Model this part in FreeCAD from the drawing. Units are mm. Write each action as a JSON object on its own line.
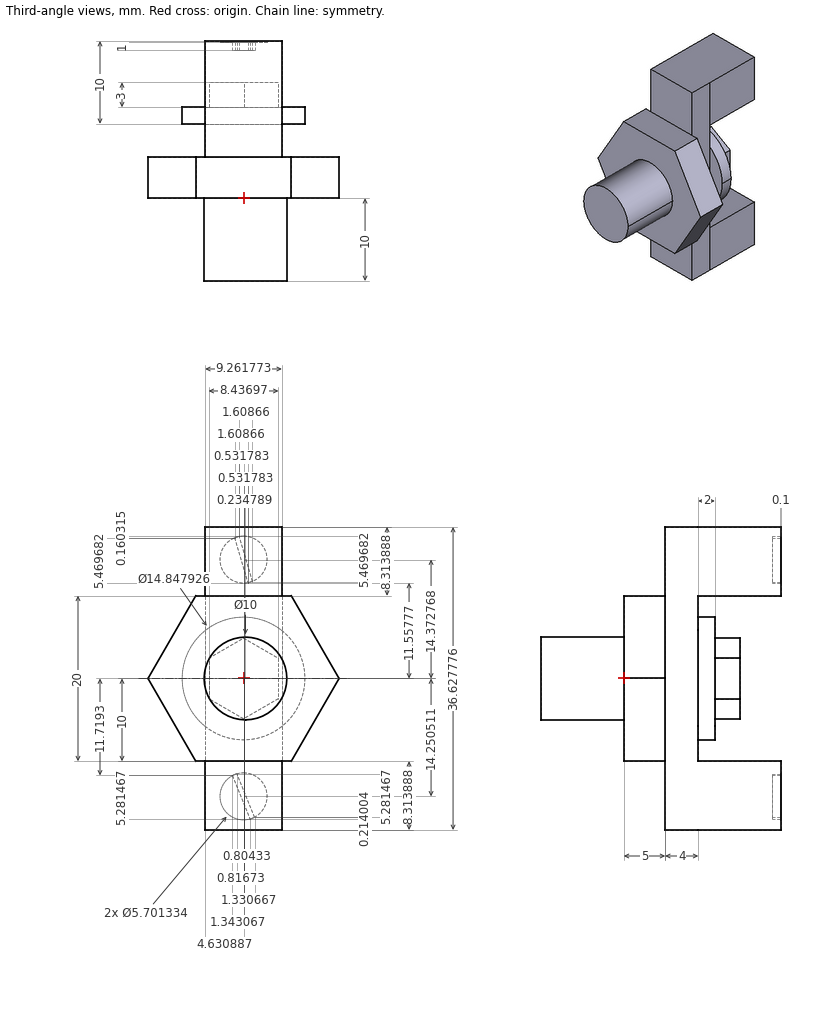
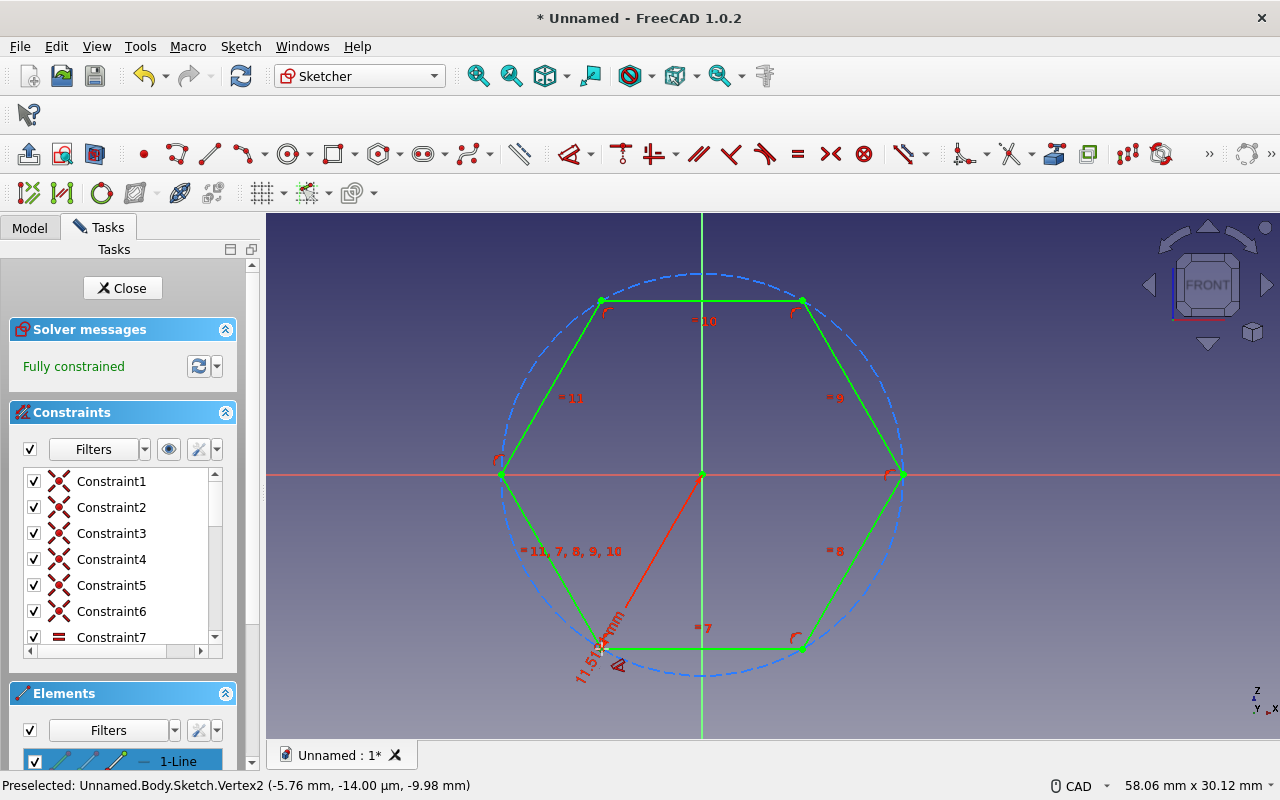
{"action": "left_click", "coordinate": [803, 301]}
{"action": "left_click", "coordinate": [837, 395]}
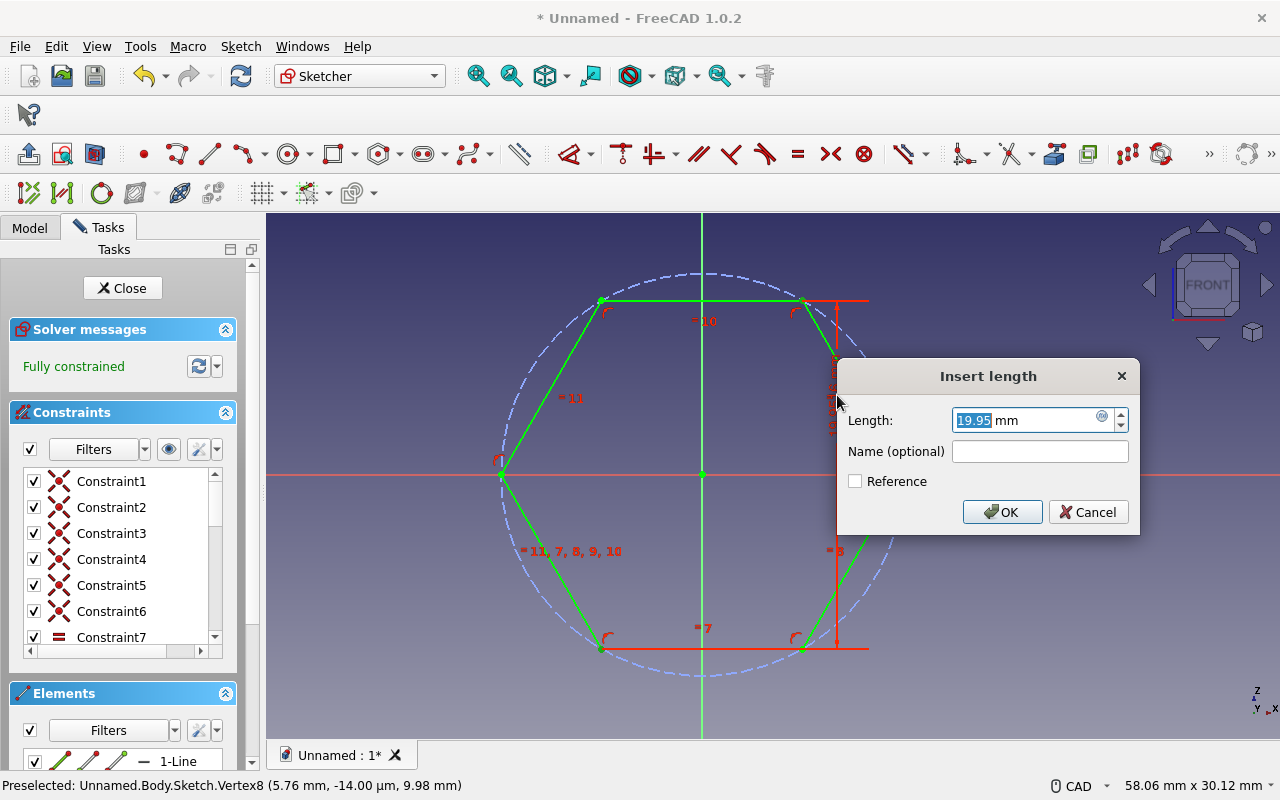
{"action": "type", "text": "20"}
{"action": "key", "text": "Return"}
{"action": "key", "text": "Escape"}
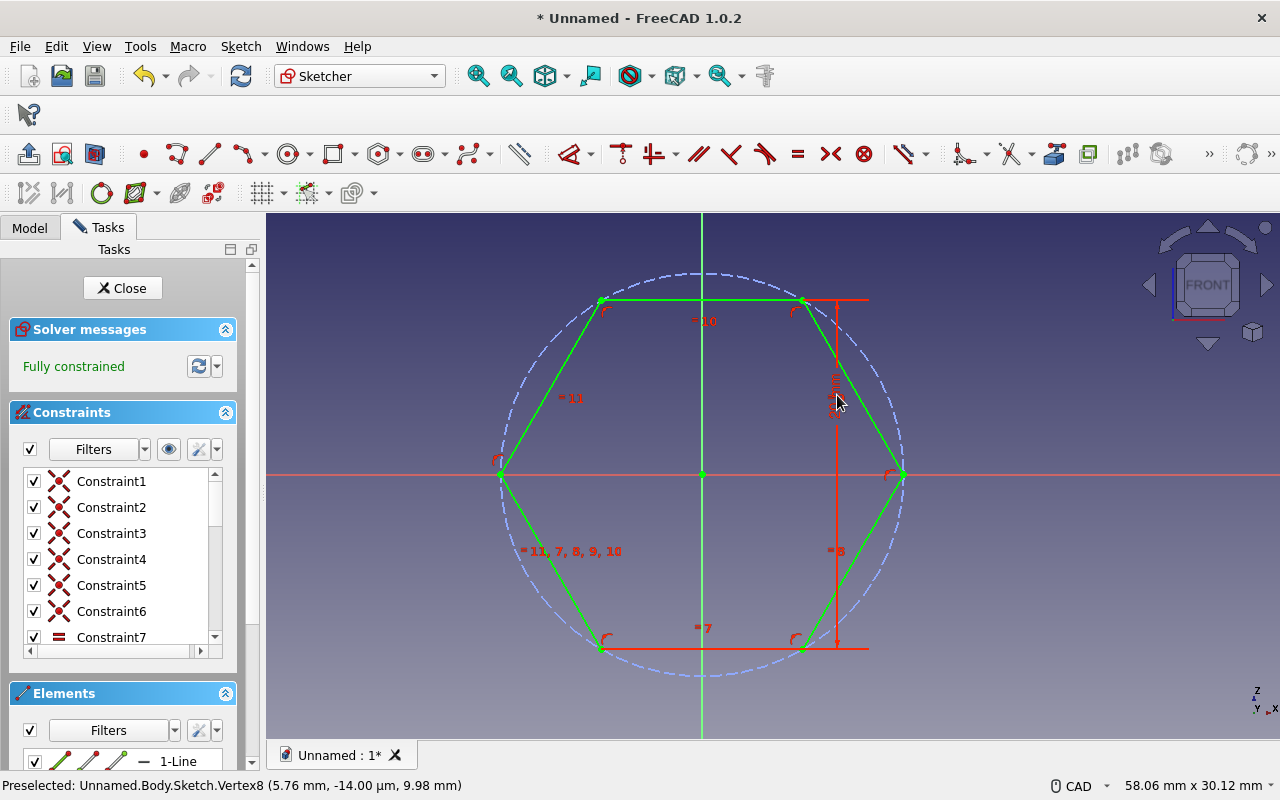
{"action": "left_click", "coordinate": [123, 288]}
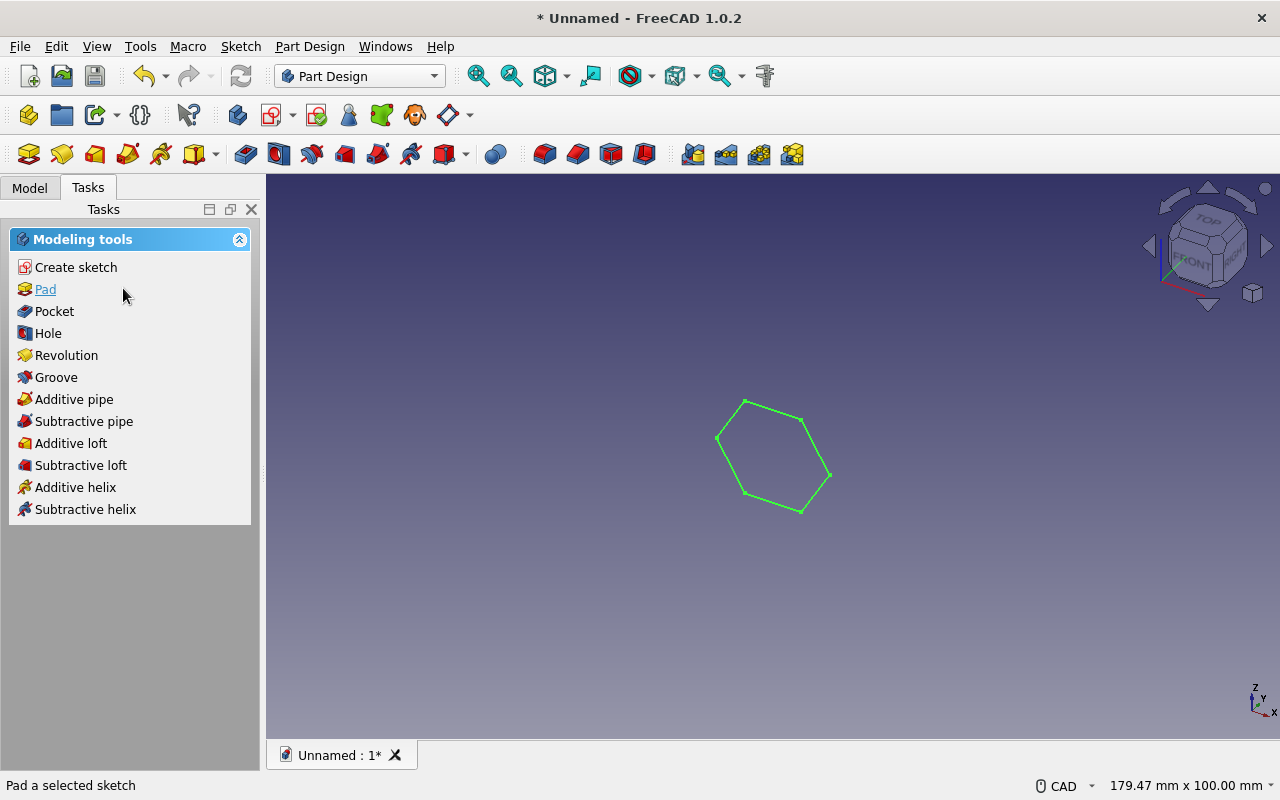
{"action": "left_click", "coordinate": [29, 154]}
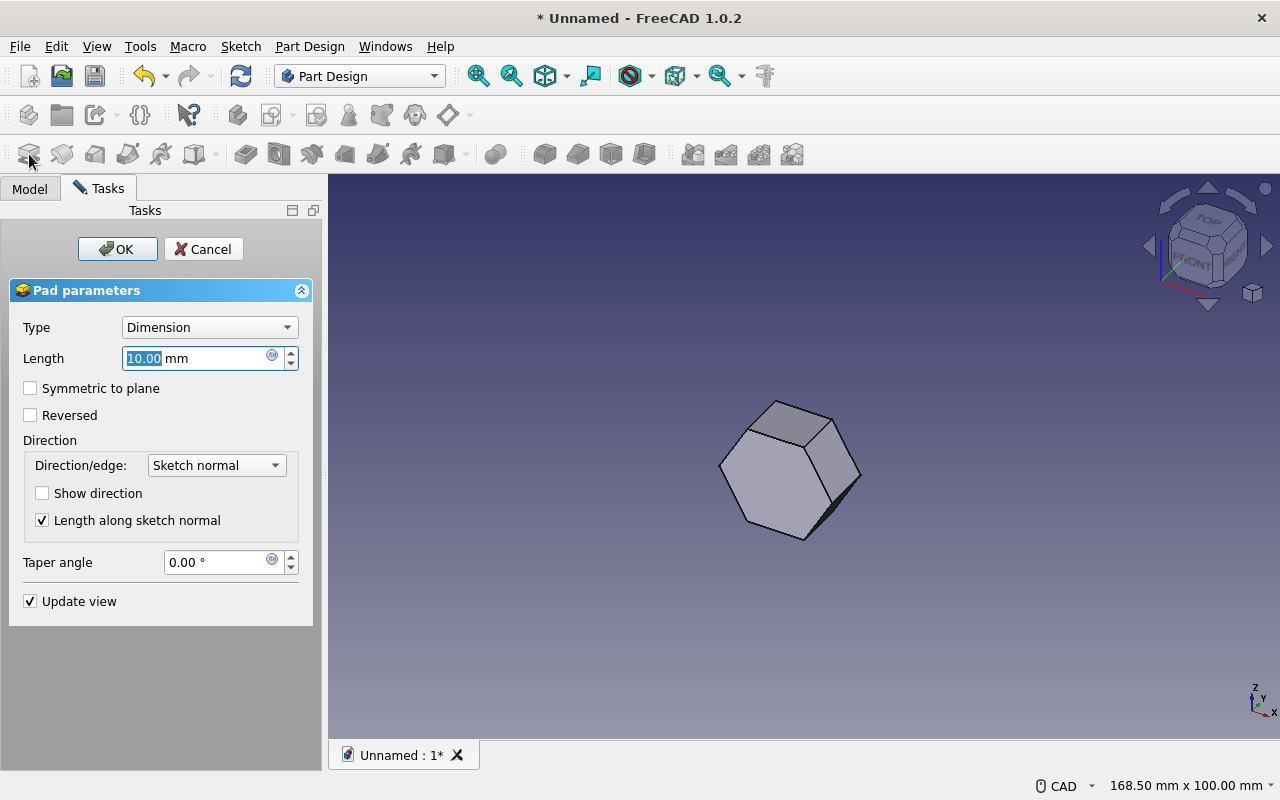
{"action": "type", "text": "5"}
{"action": "key", "text": "Tab"}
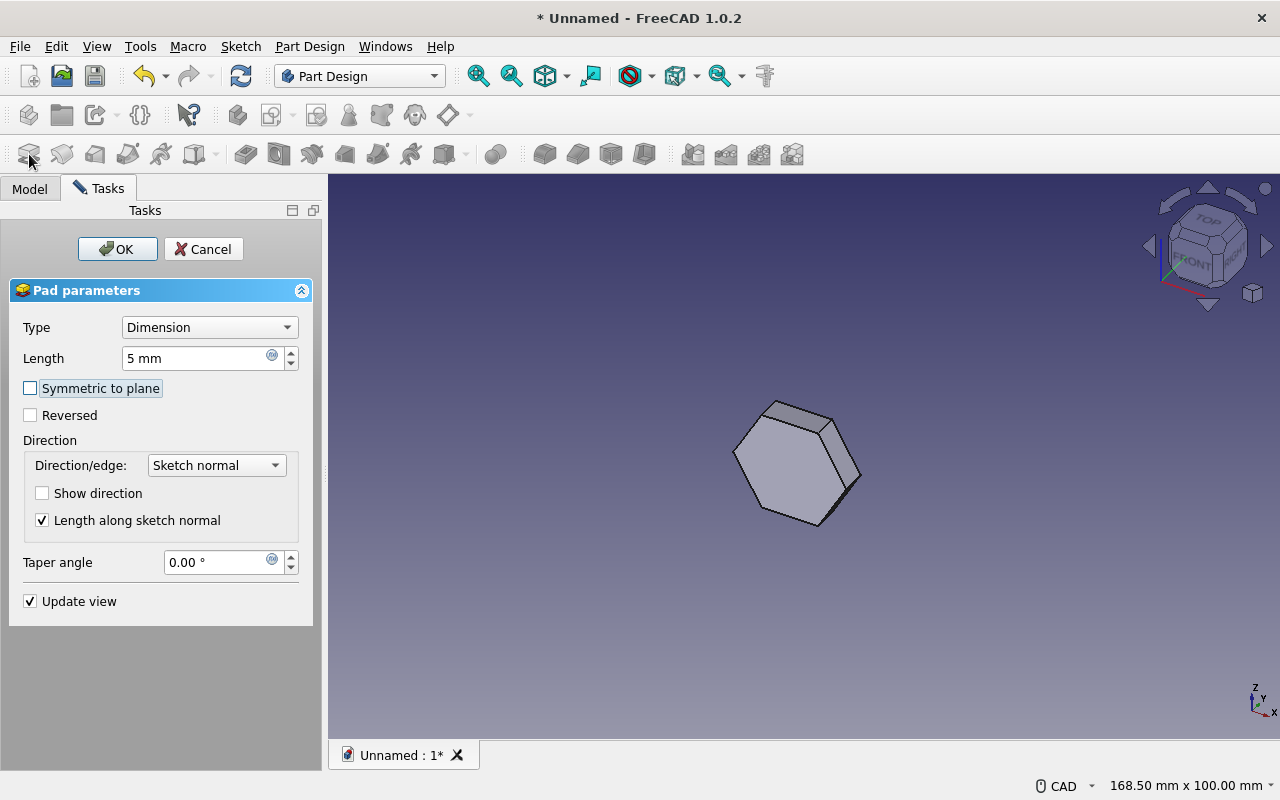
{"action": "left_click", "coordinate": [31, 415]}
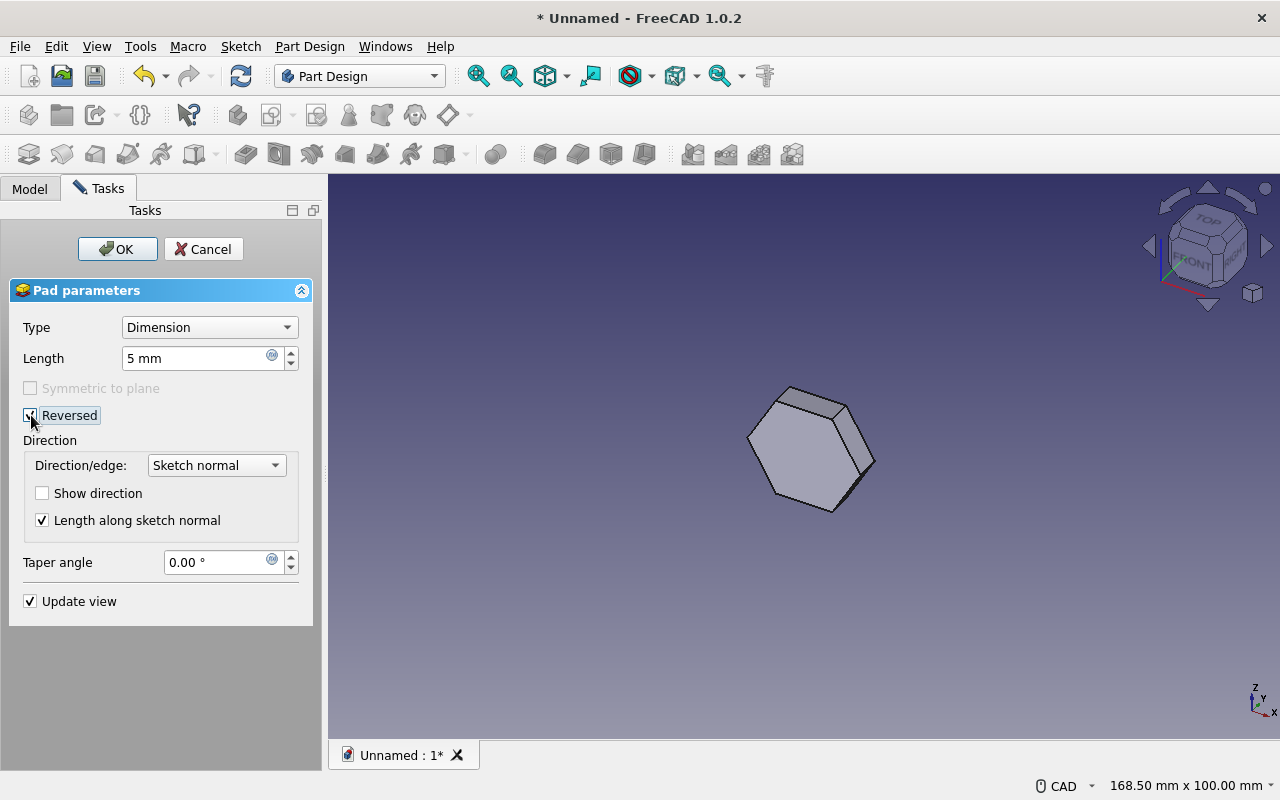
{"action": "left_click", "coordinate": [118, 249]}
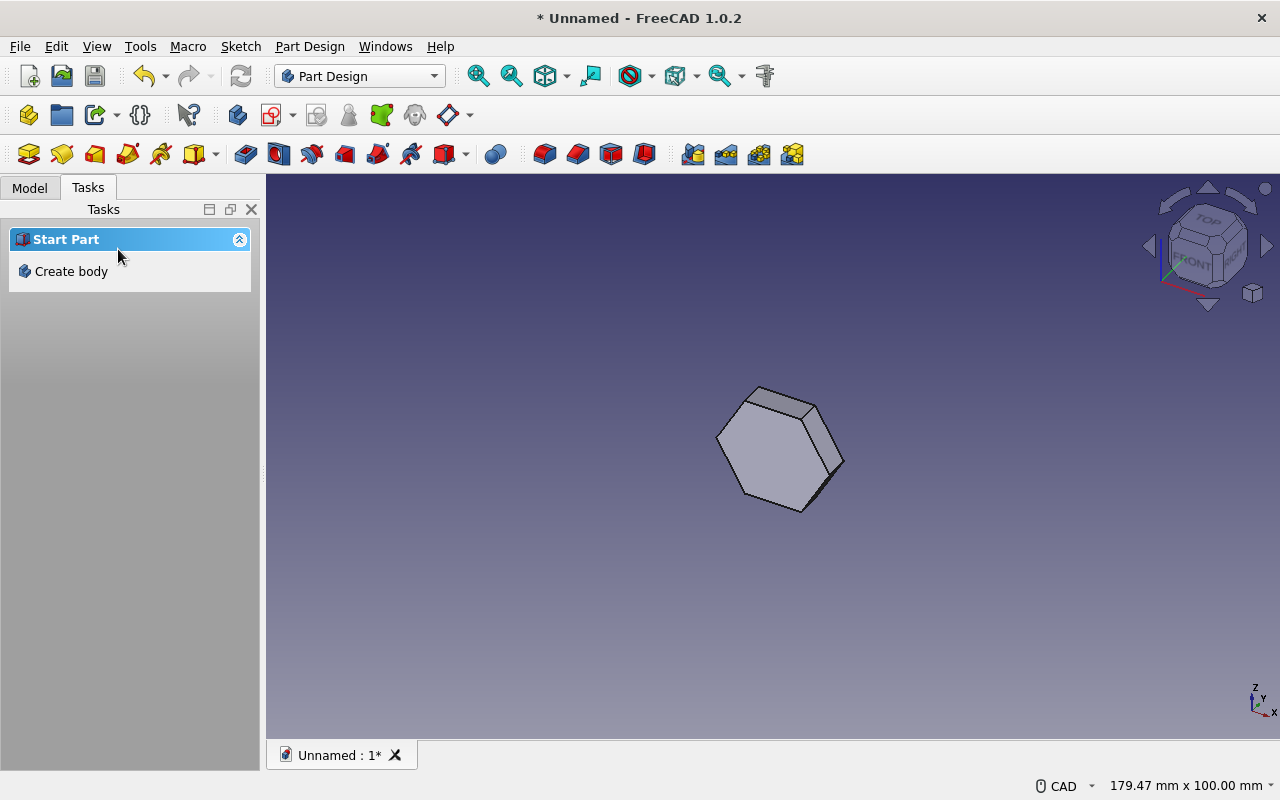
{"action": "left_click", "coordinate": [479, 76]}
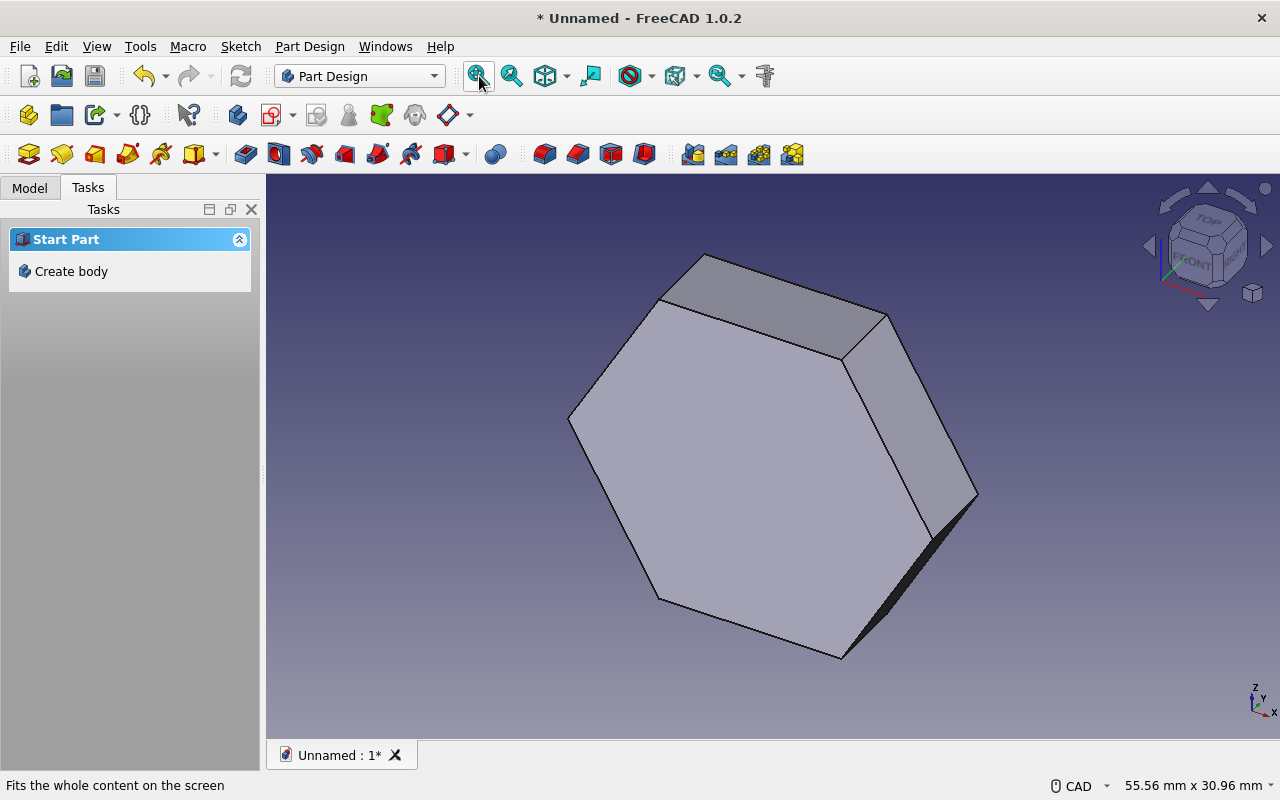
{"action": "left_click", "coordinate": [270, 116]}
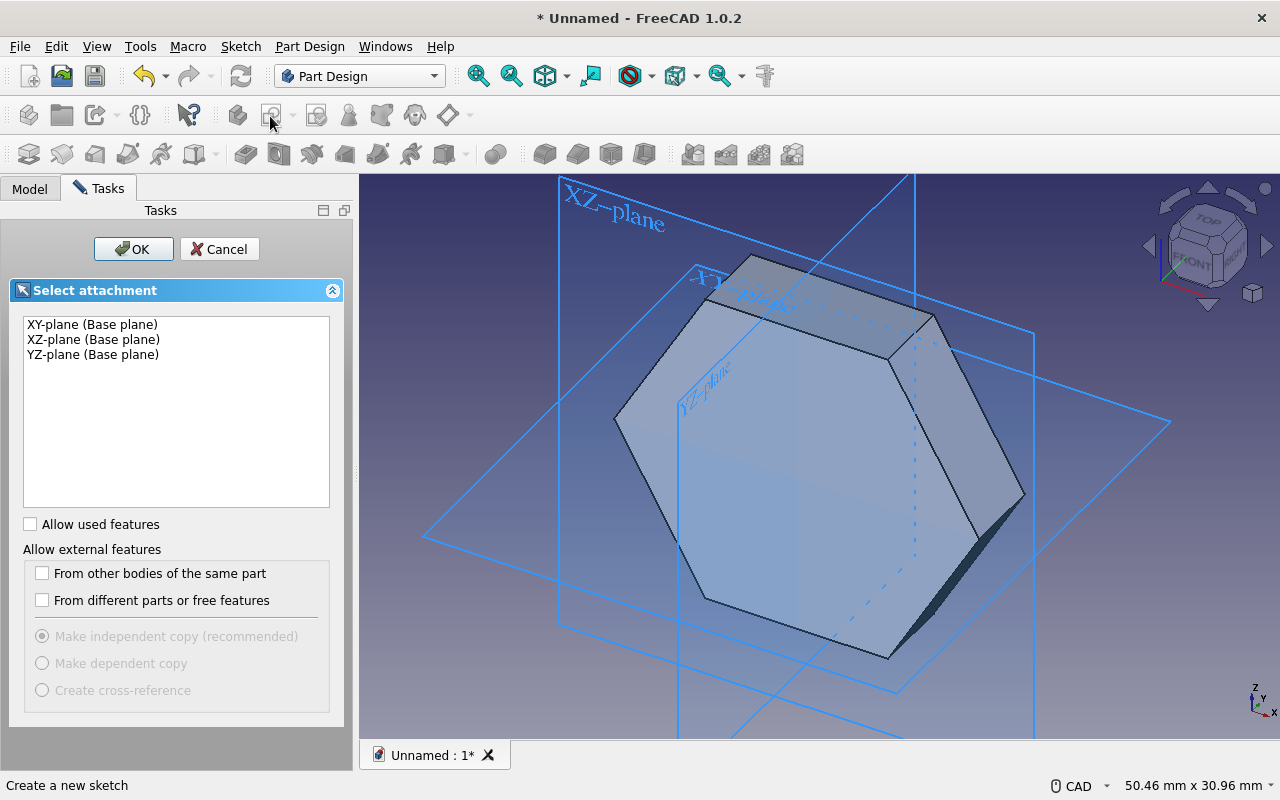
{"action": "left_click", "coordinate": [84, 340]}